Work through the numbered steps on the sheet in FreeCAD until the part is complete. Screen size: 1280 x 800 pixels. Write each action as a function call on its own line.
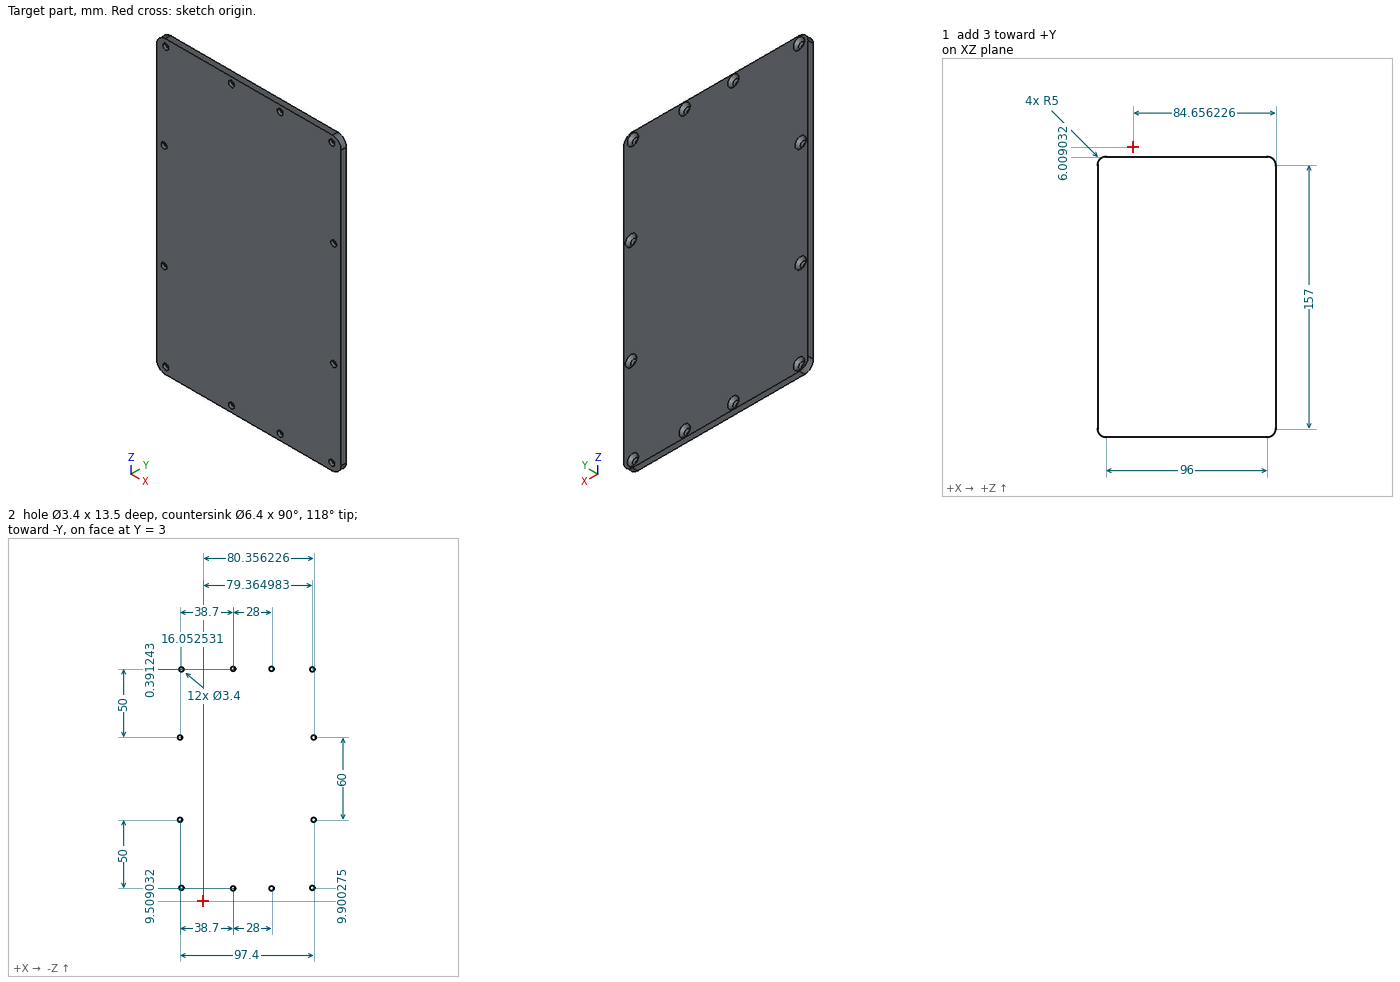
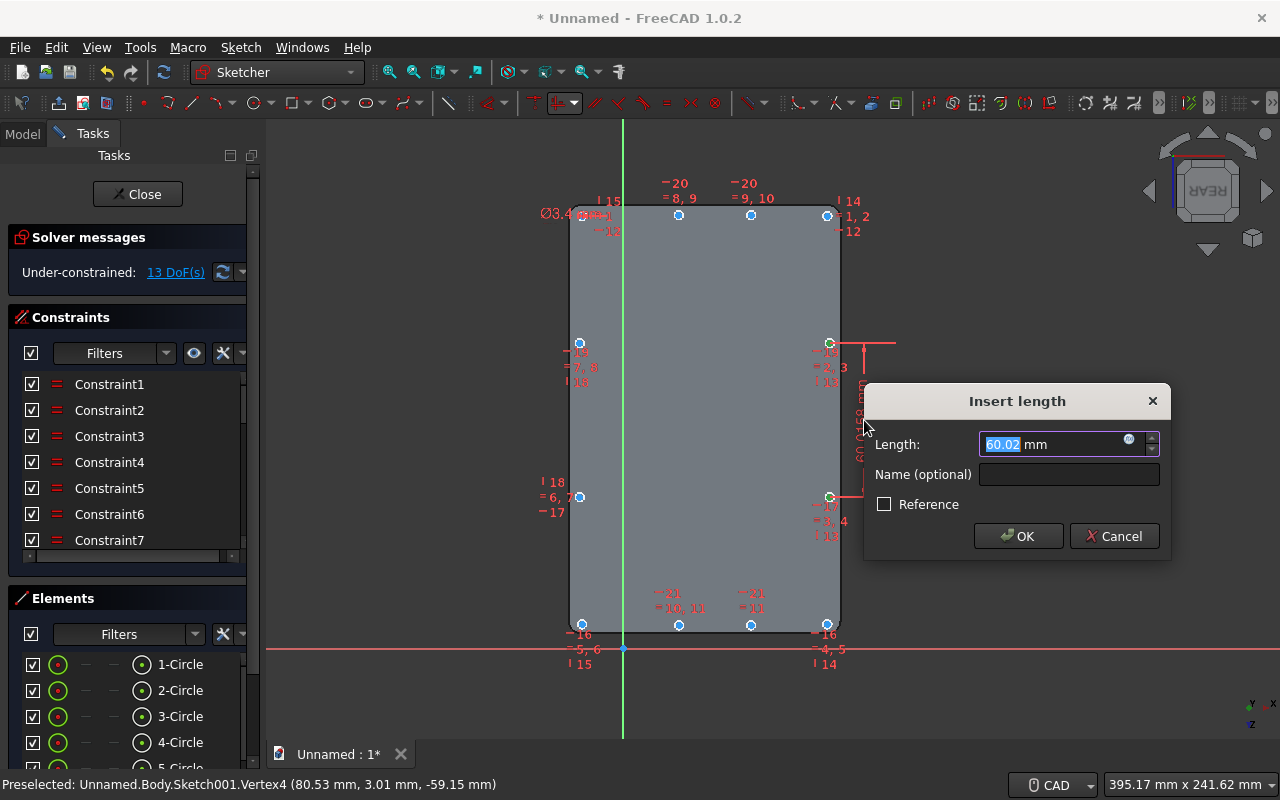
text(60)
key(Return)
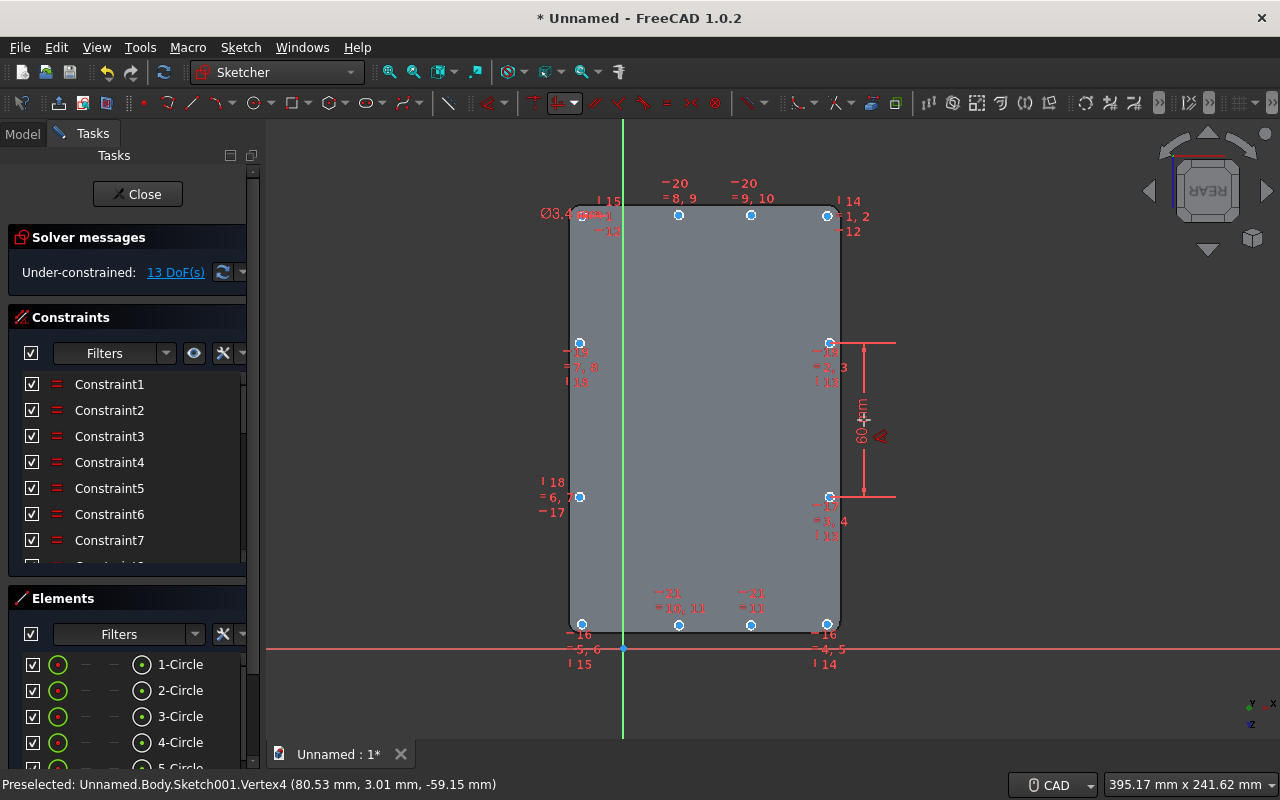
click(580, 343)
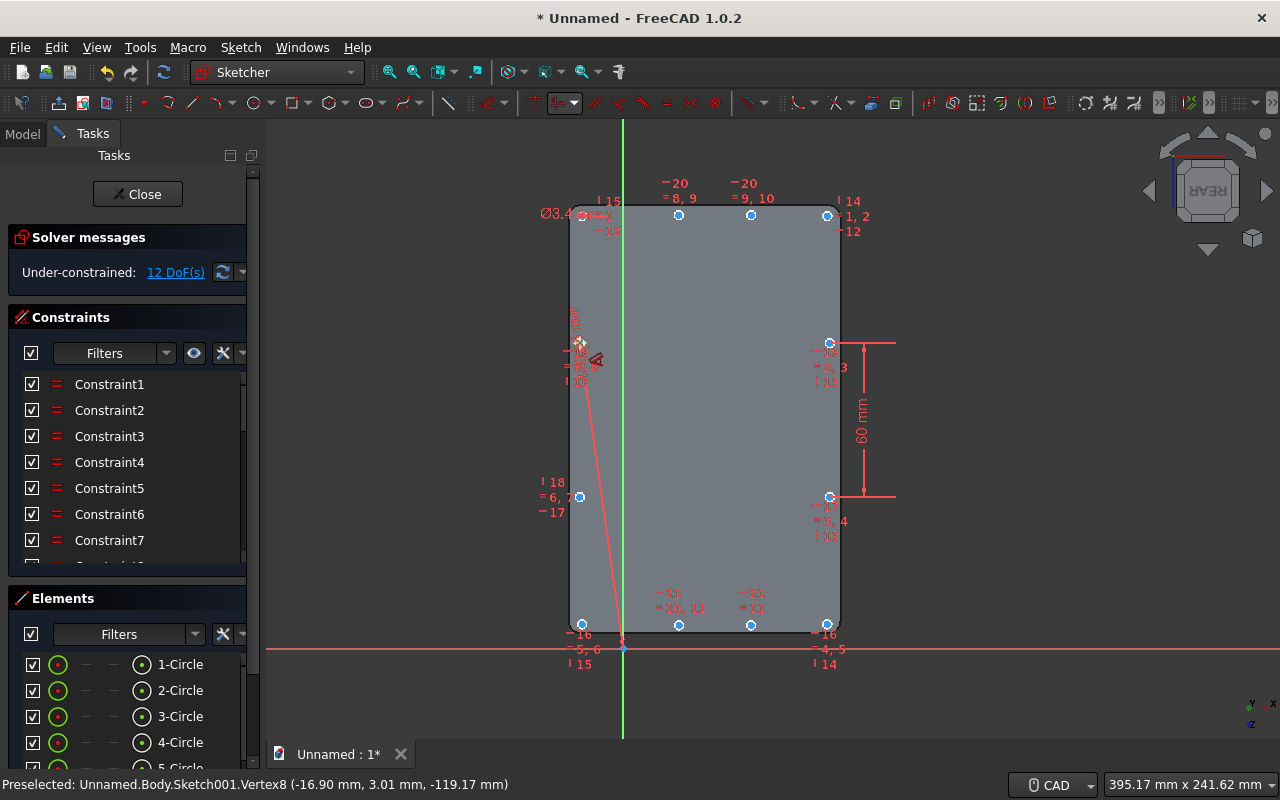
click(679, 215)
click(546, 279)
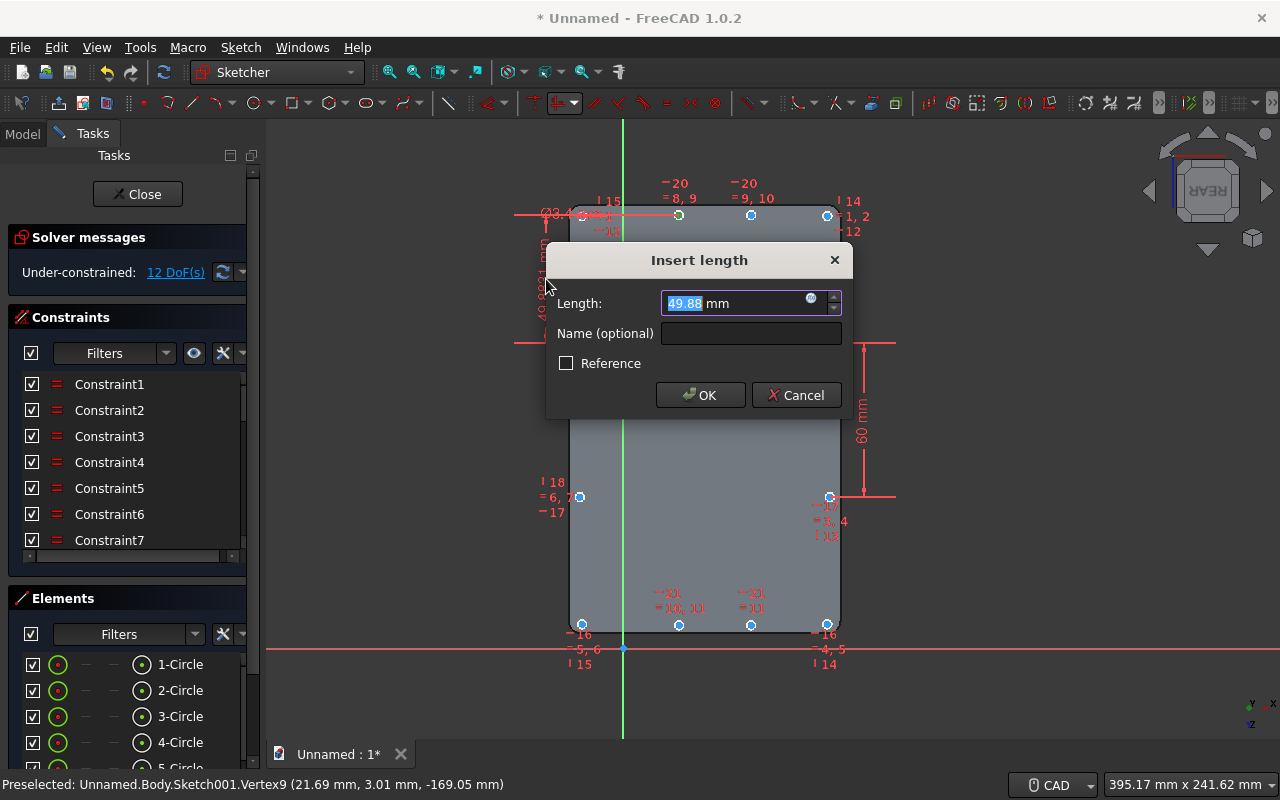
text(50)
key(Return)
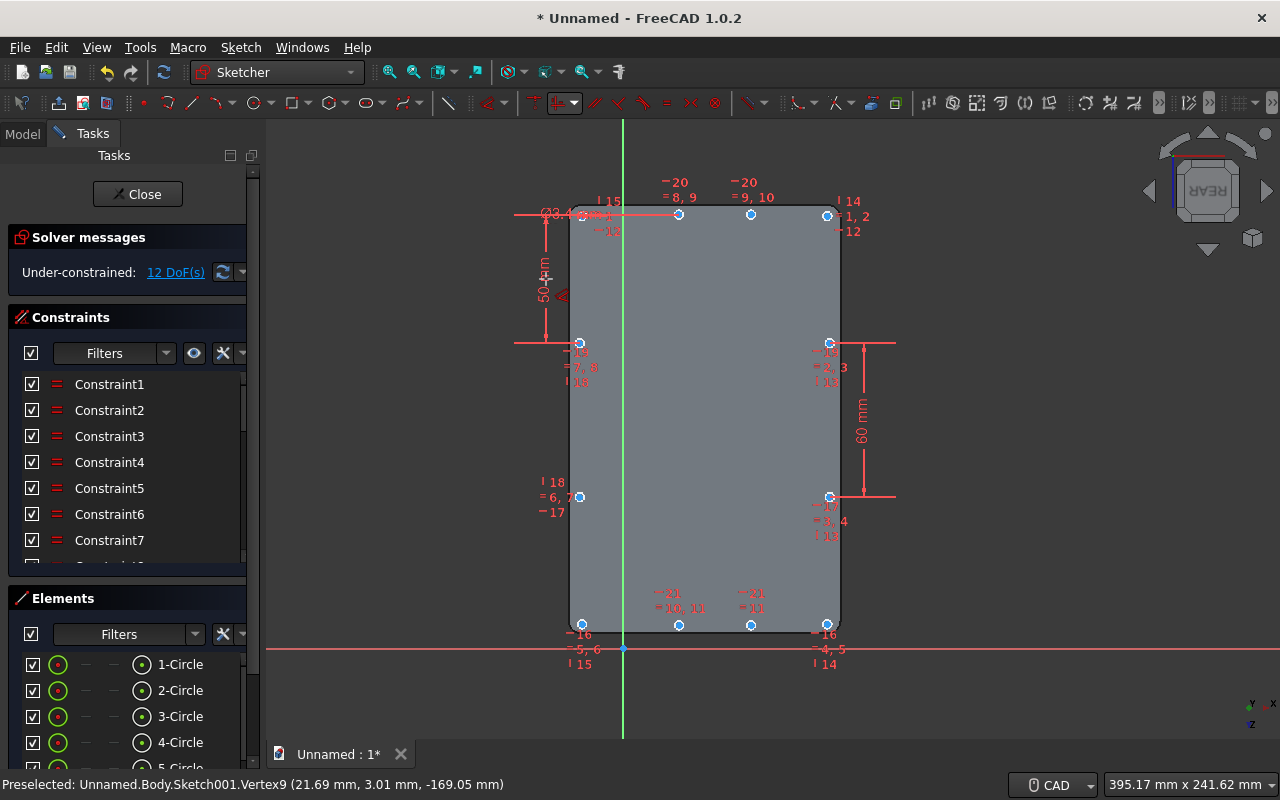
click(679, 215)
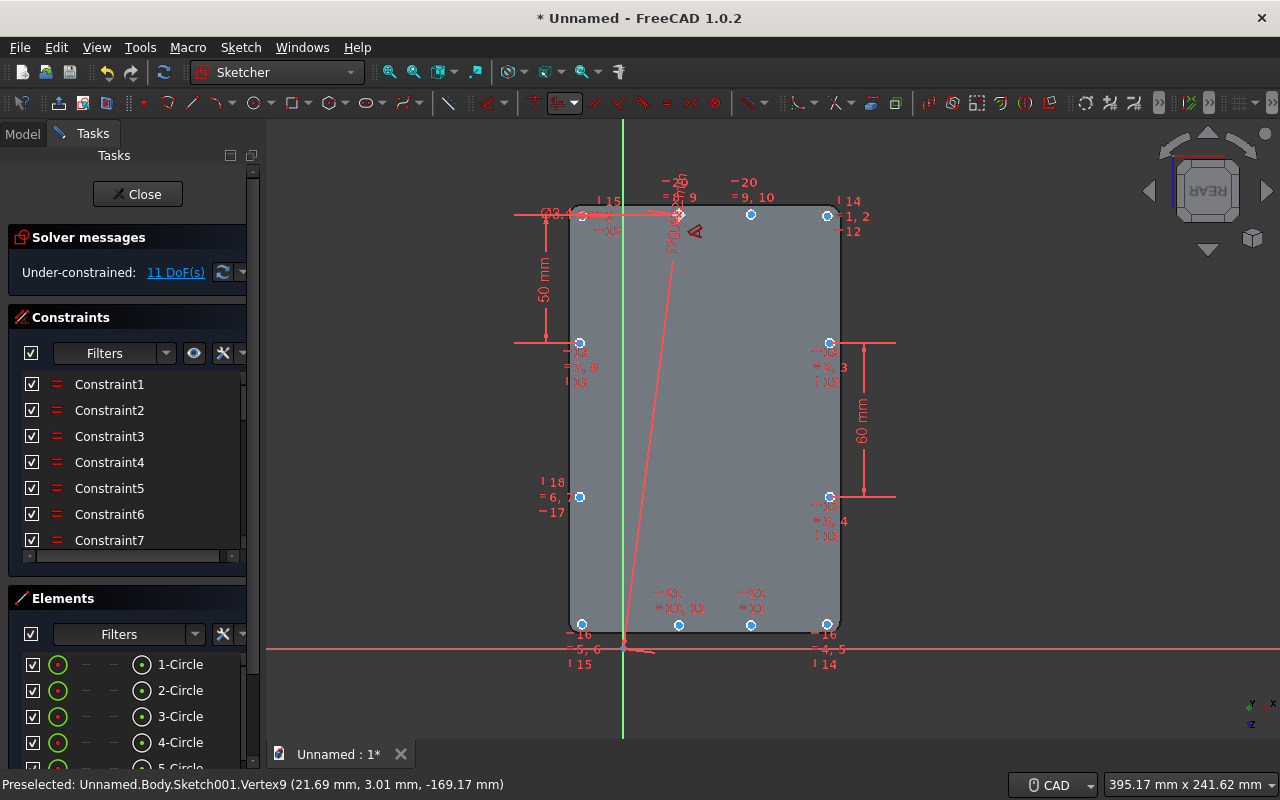
click(751, 215)
click(715, 181)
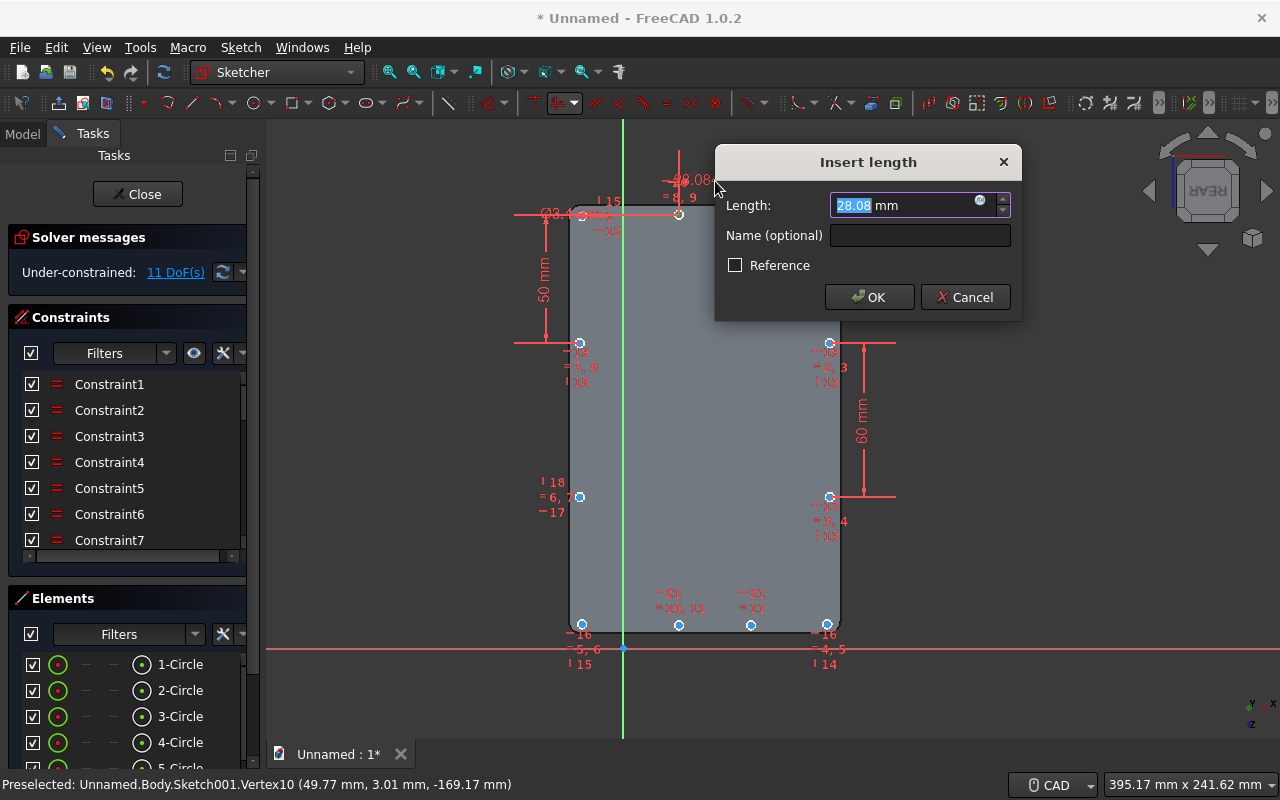
text(28)
key(Return)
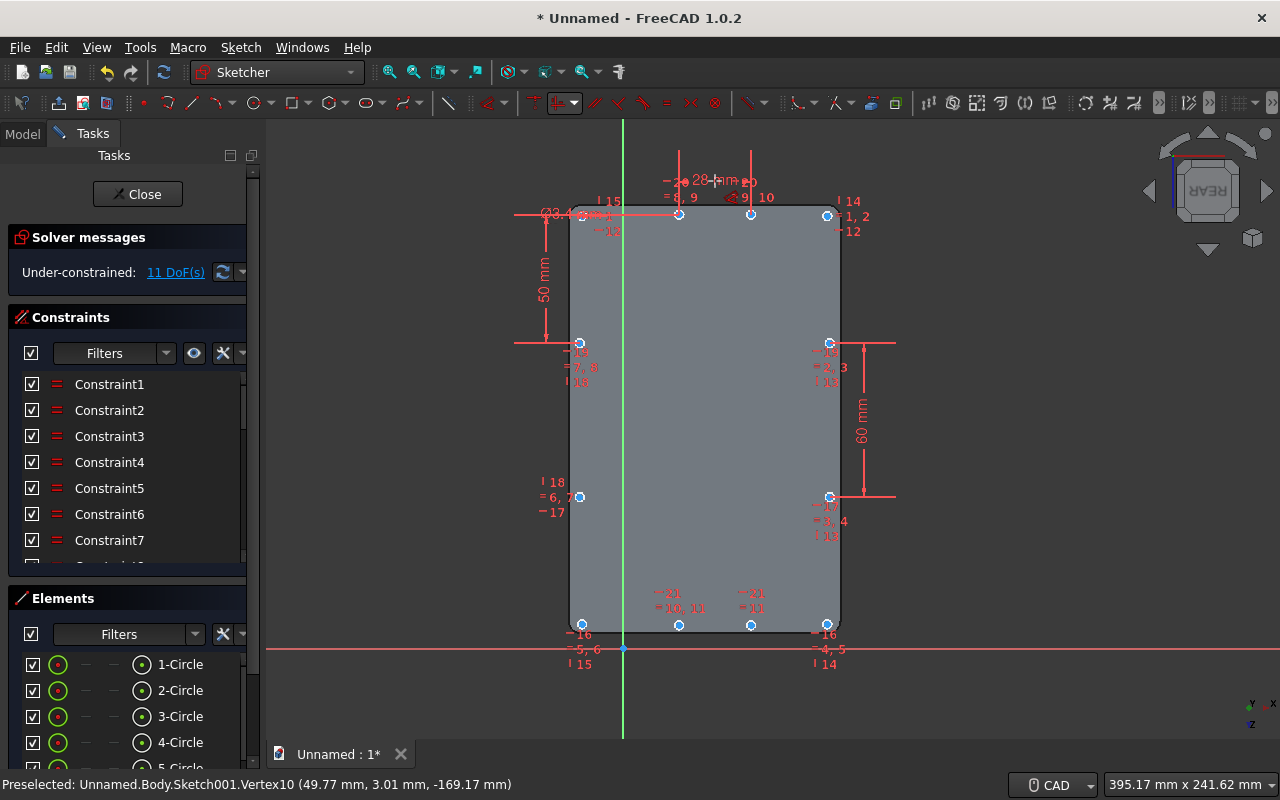
click(580, 497)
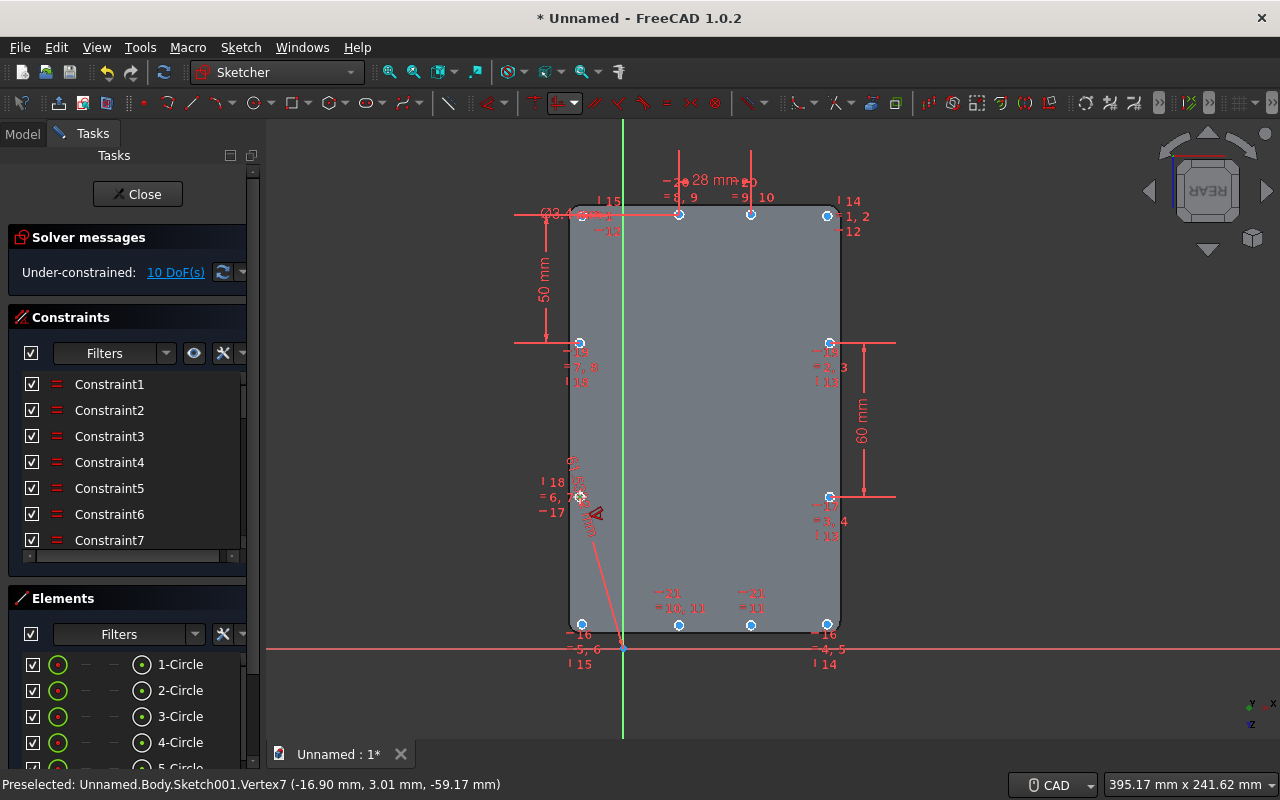
click(679, 625)
click(546, 561)